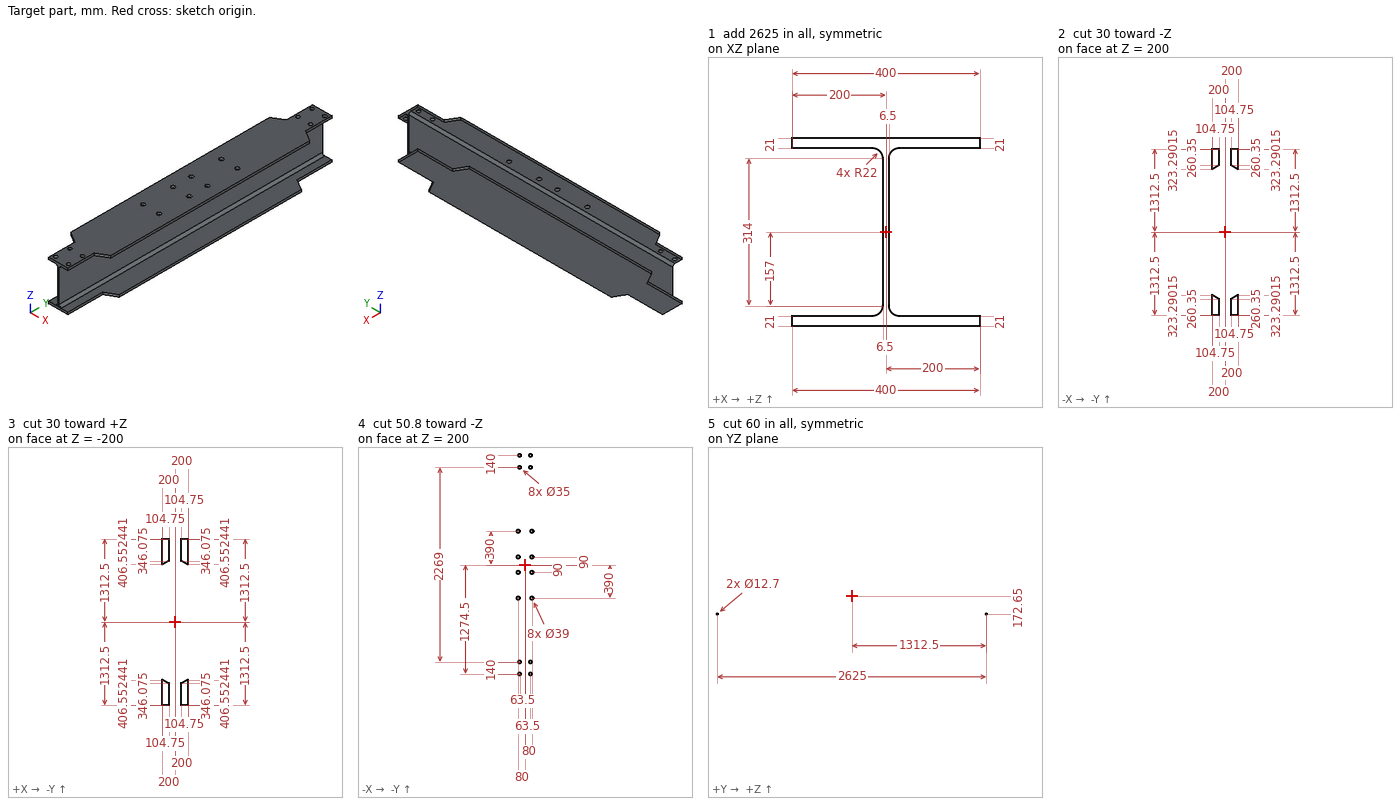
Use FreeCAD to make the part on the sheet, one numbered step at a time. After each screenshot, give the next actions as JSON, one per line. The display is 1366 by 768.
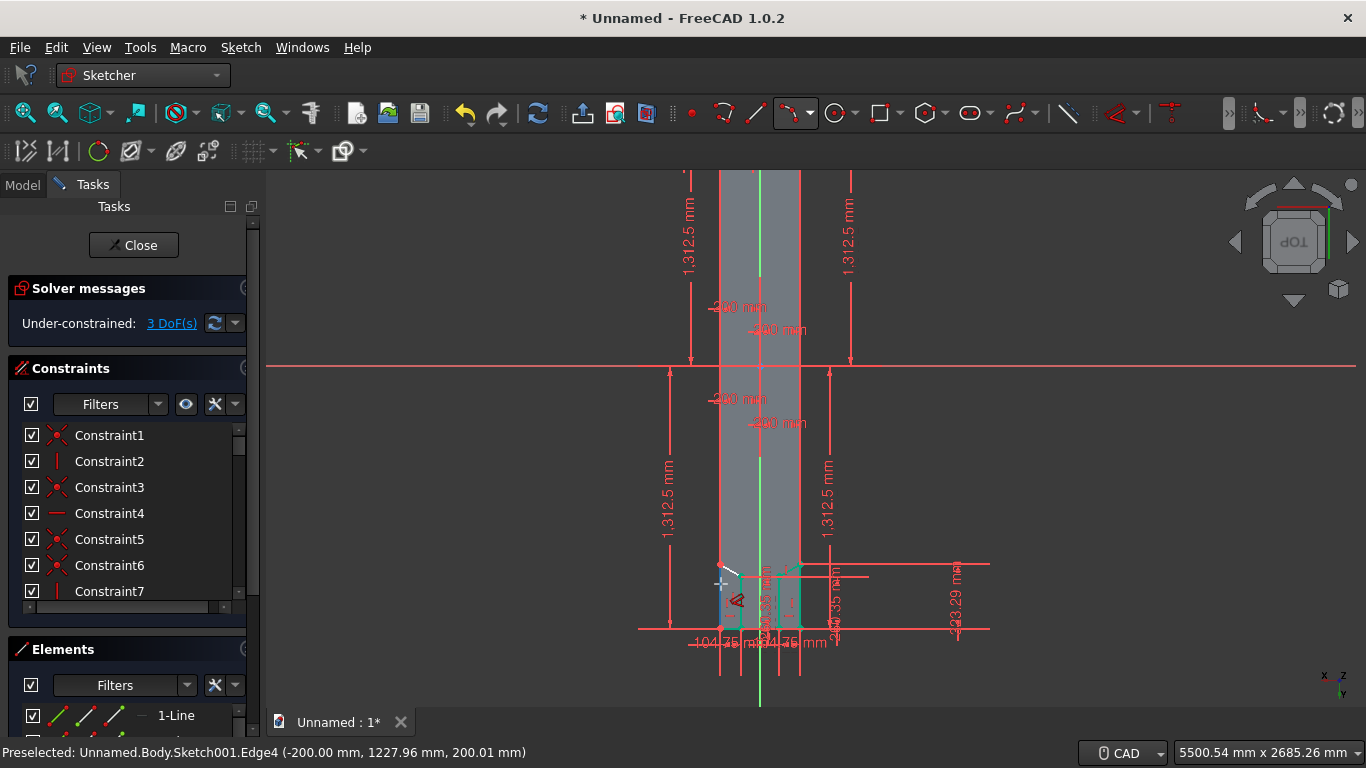
{"action": "left_click", "coordinate": [720, 584]}
{"action": "left_click", "coordinate": [686, 597]}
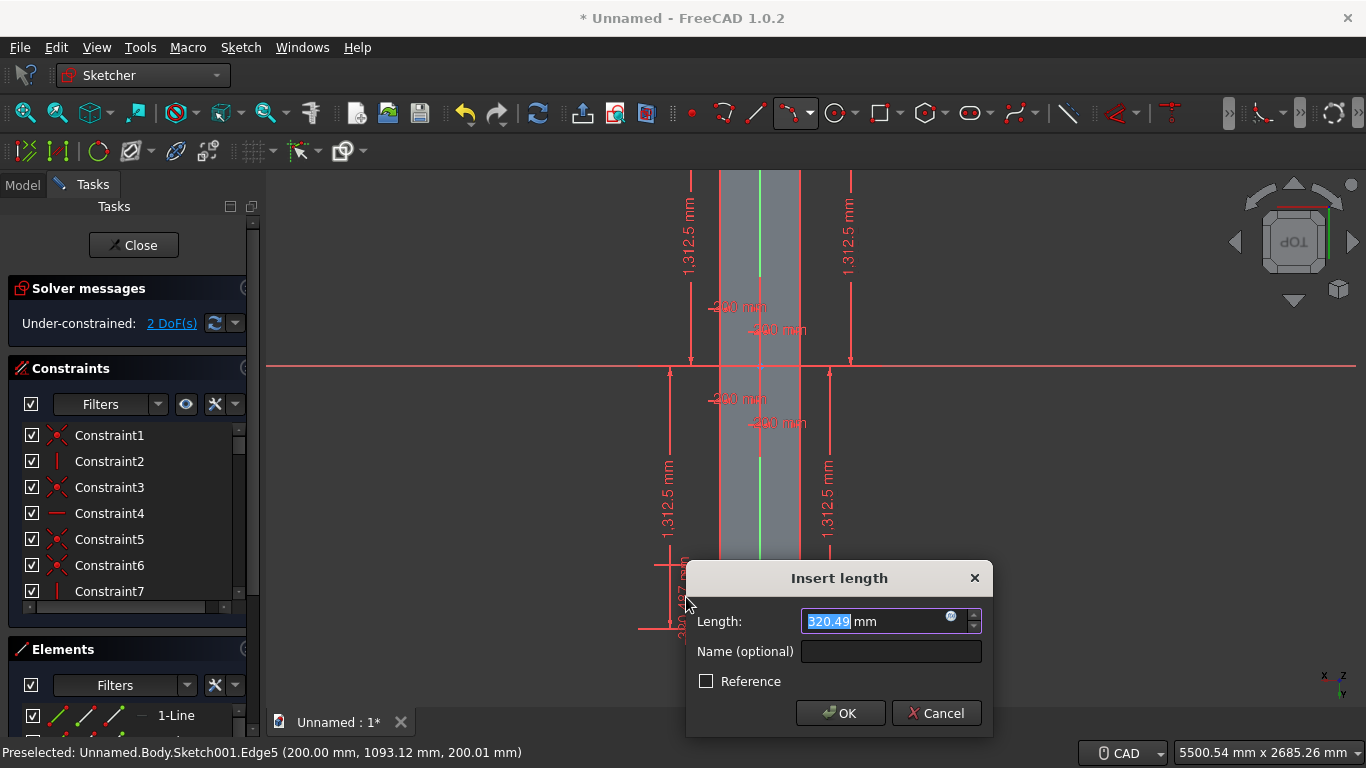
{"action": "type", "text": "323.29015"}
{"action": "key", "text": "Return"}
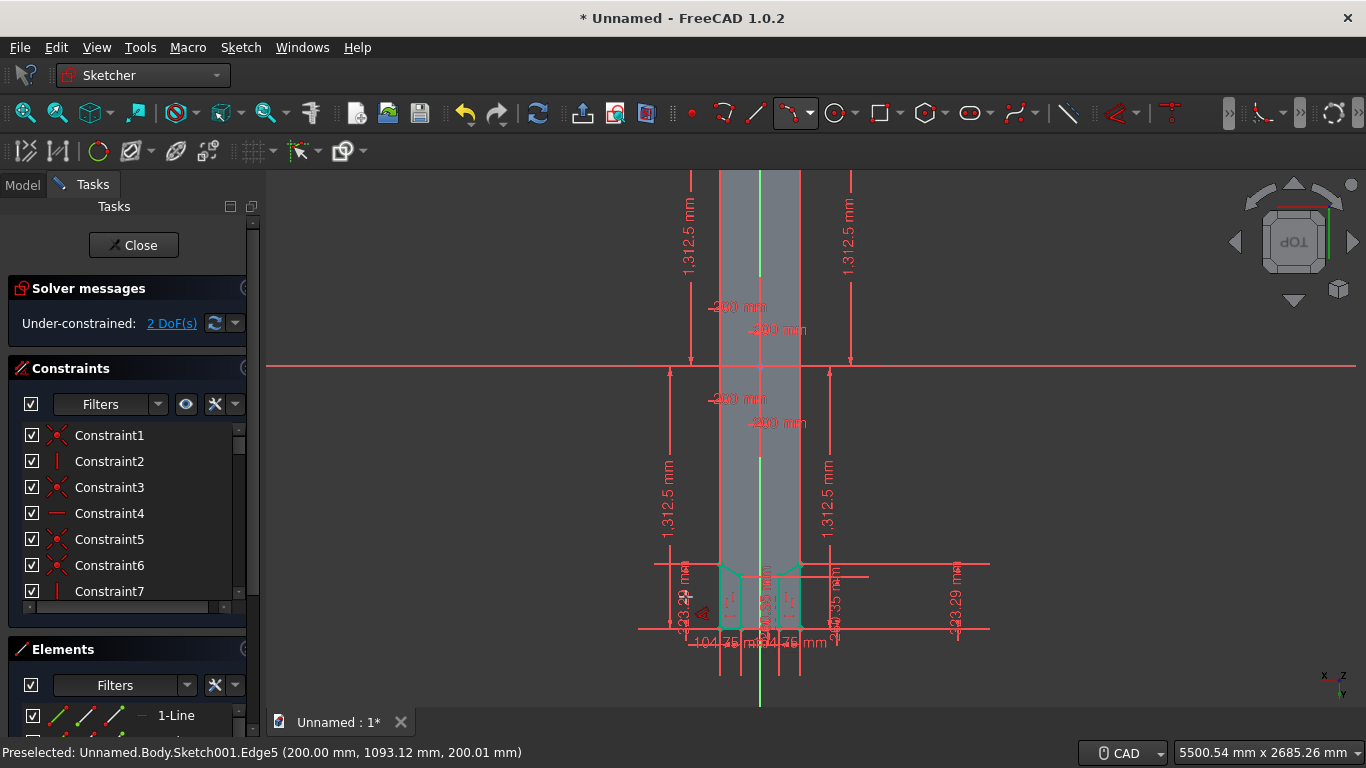
{"action": "scroll", "coordinate": [721, 585], "scroll_direction": "down", "scroll_amount": 2}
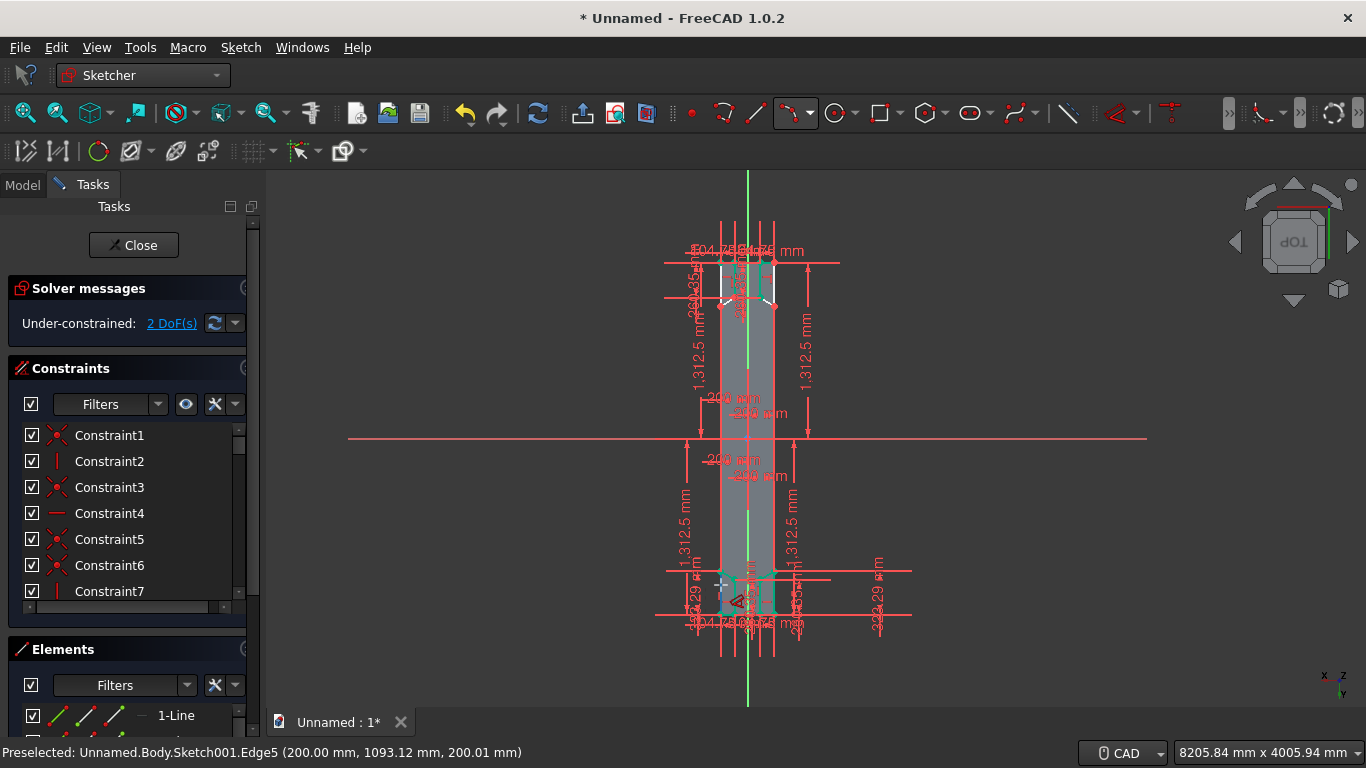
{"action": "left_click", "coordinate": [721, 276]}
{"action": "left_click", "coordinate": [615, 285]}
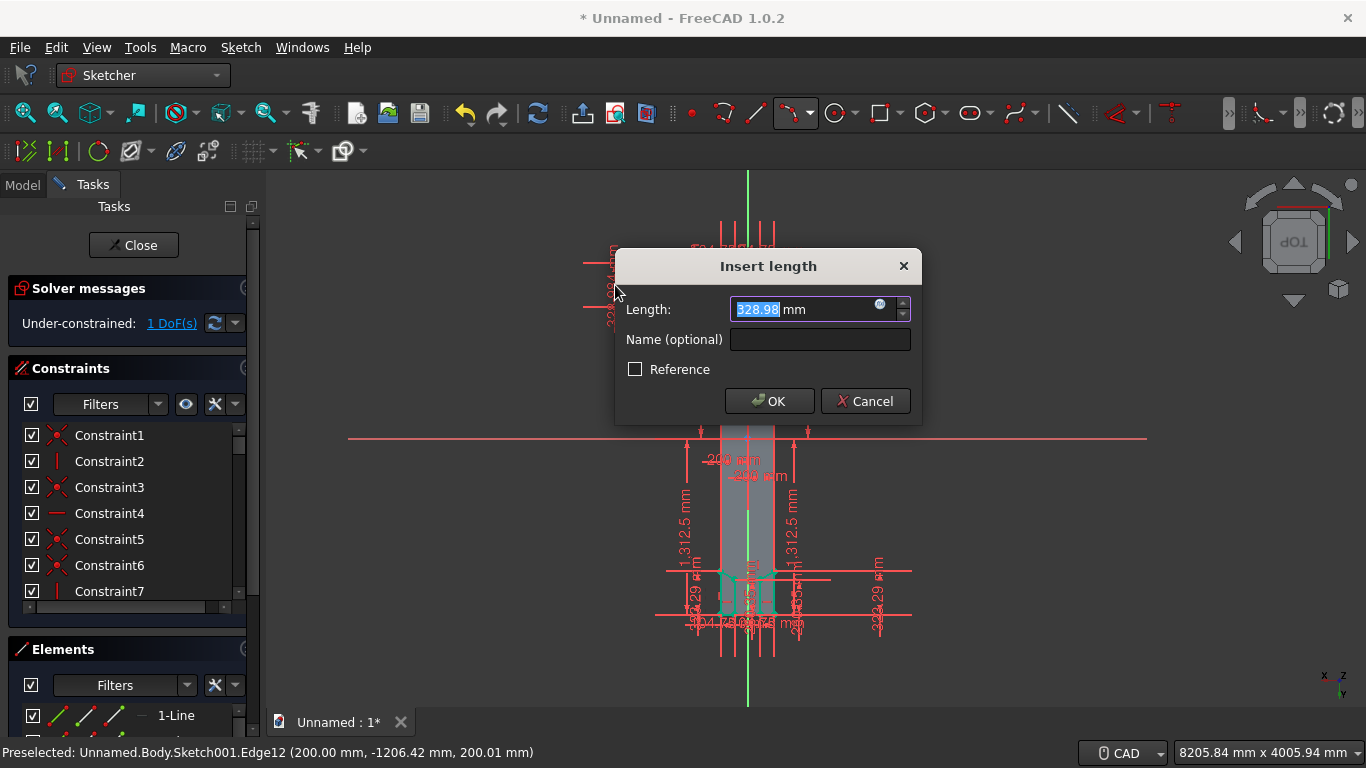
{"action": "type", "text": "323.29015"}
{"action": "key", "text": "Return"}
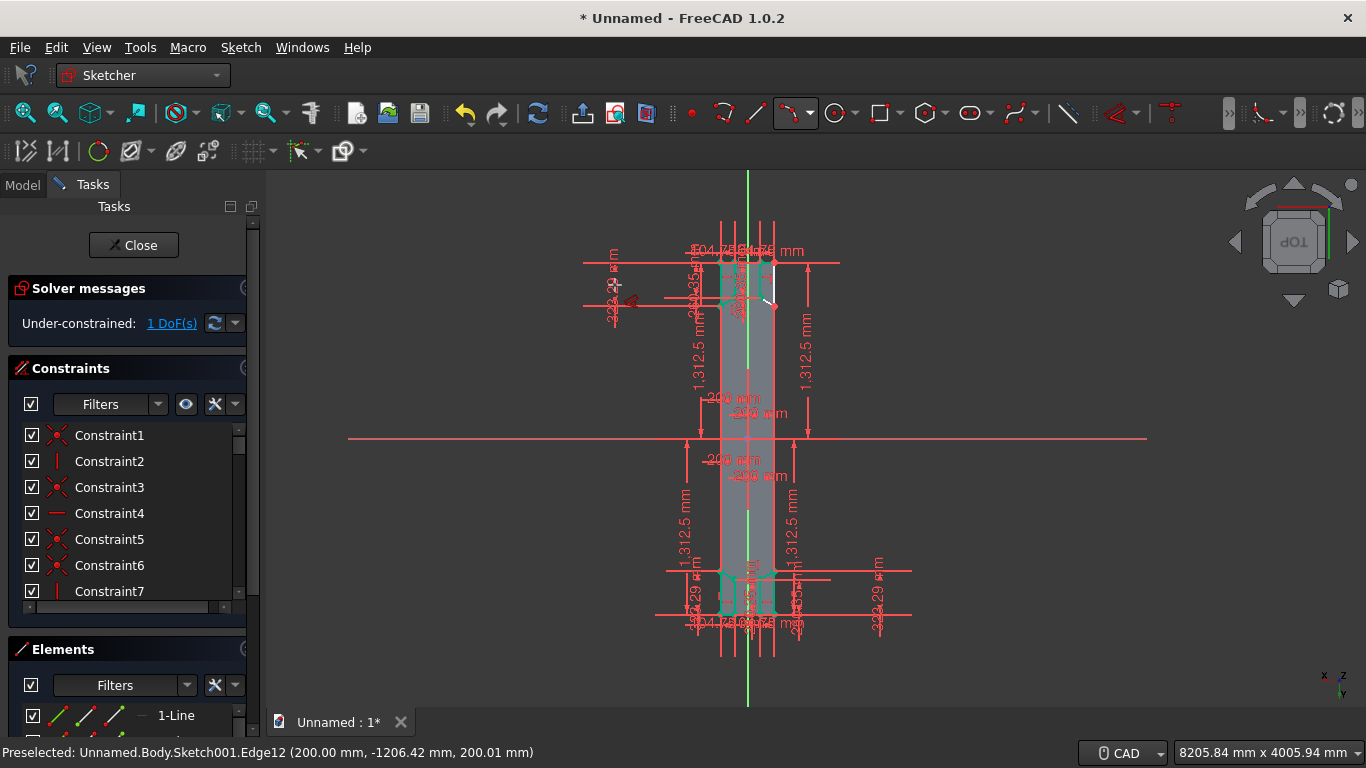
{"action": "scroll", "coordinate": [774, 293], "scroll_direction": "up", "scroll_amount": 2}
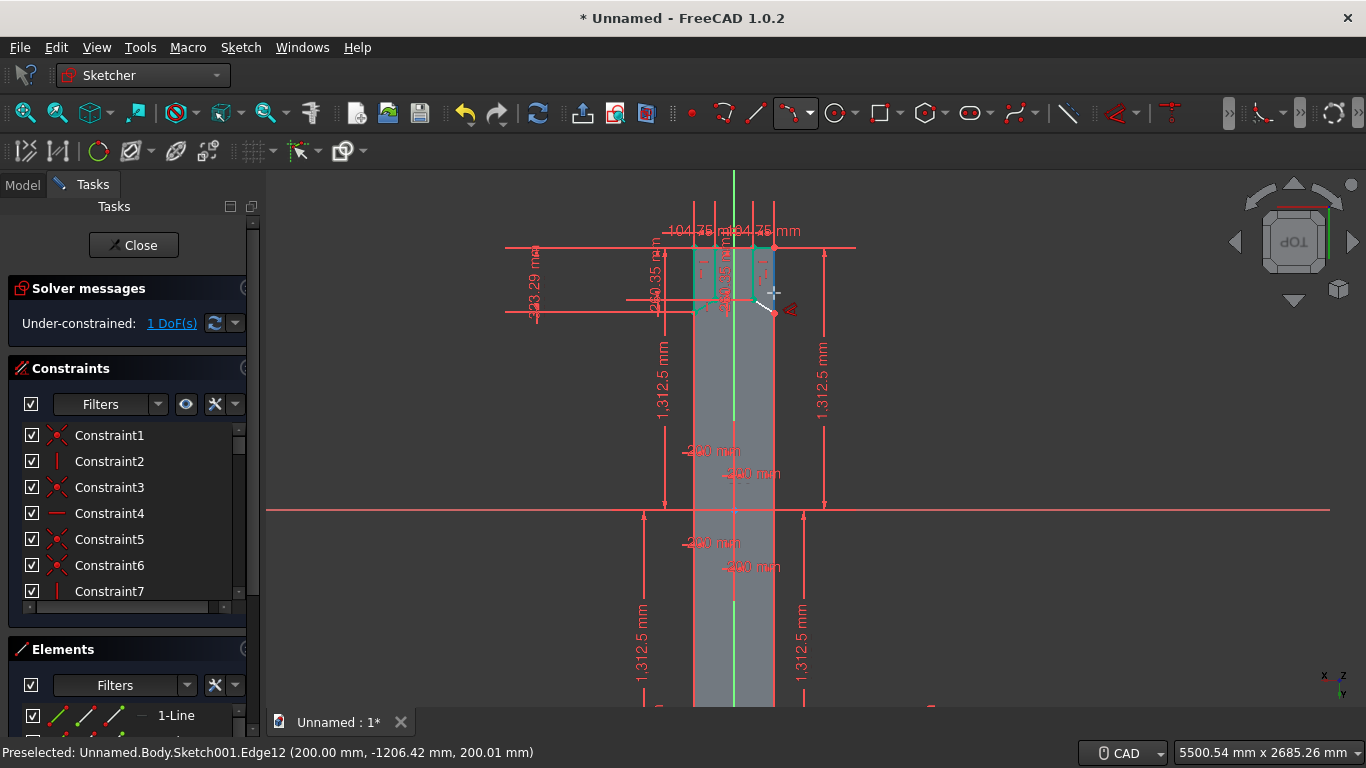
{"action": "left_click", "coordinate": [774, 293]}
{"action": "left_click", "coordinate": [808, 280]}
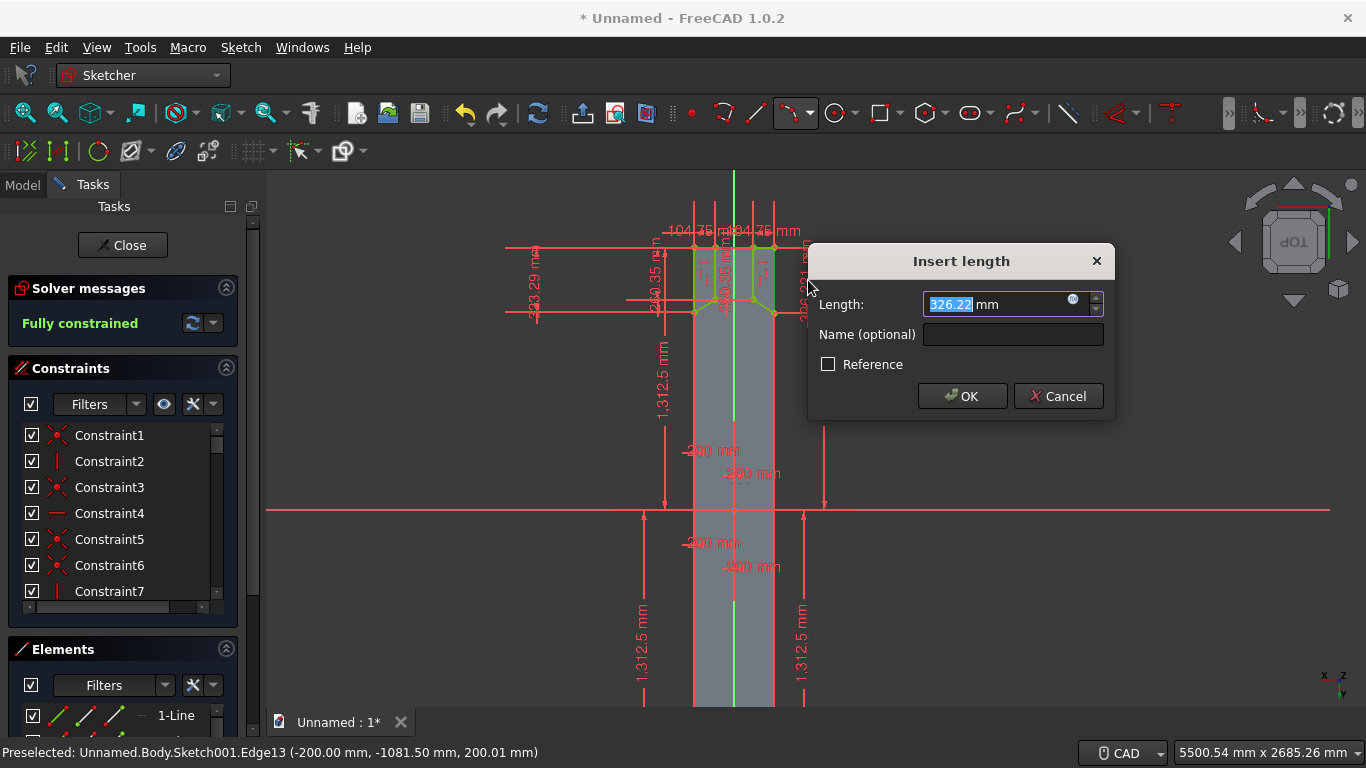
{"action": "type", "text": "323.29015"}
{"action": "key", "text": "Return"}
{"action": "key", "text": "Escape"}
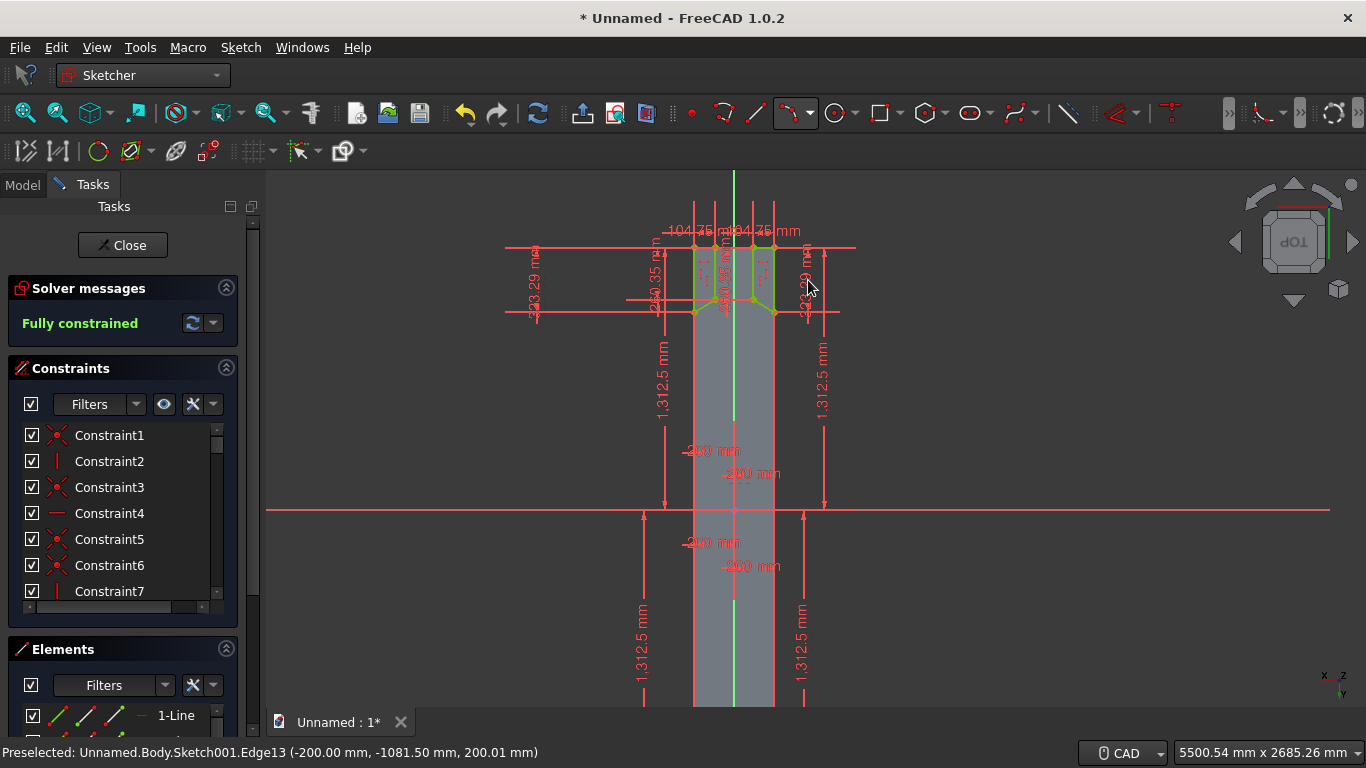
{"action": "left_click", "coordinate": [123, 245]}